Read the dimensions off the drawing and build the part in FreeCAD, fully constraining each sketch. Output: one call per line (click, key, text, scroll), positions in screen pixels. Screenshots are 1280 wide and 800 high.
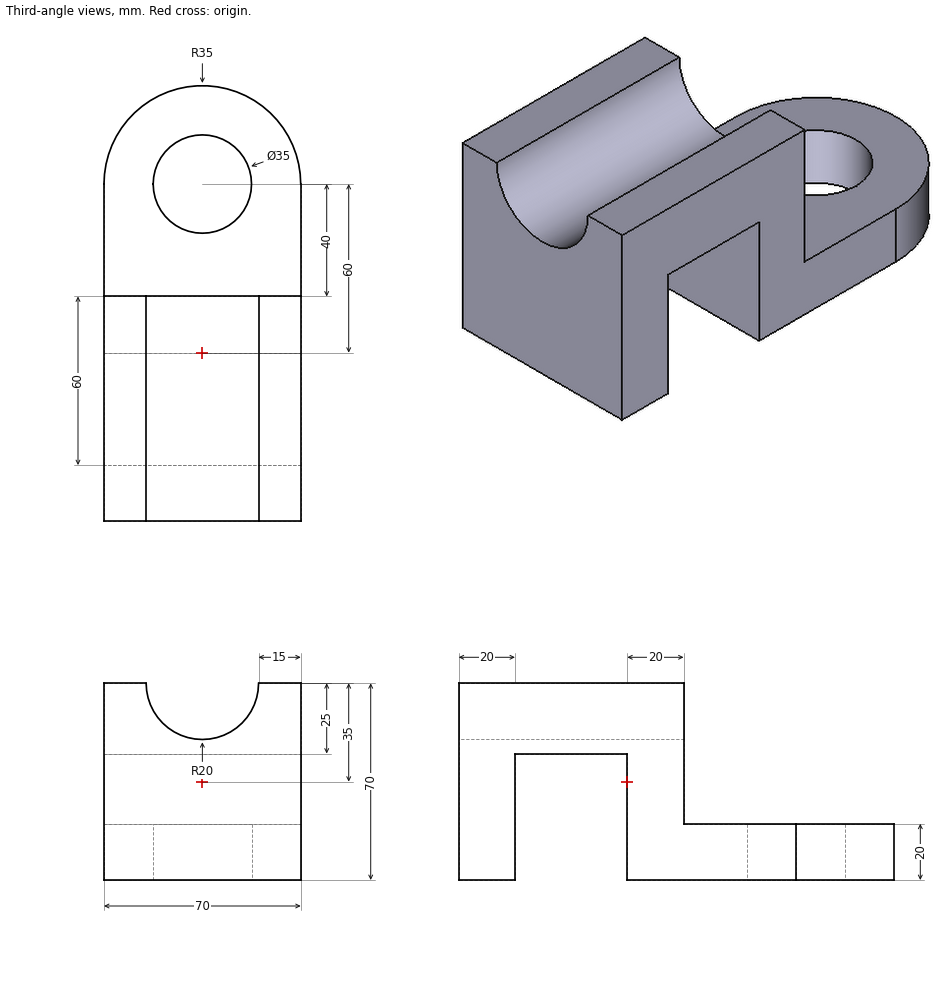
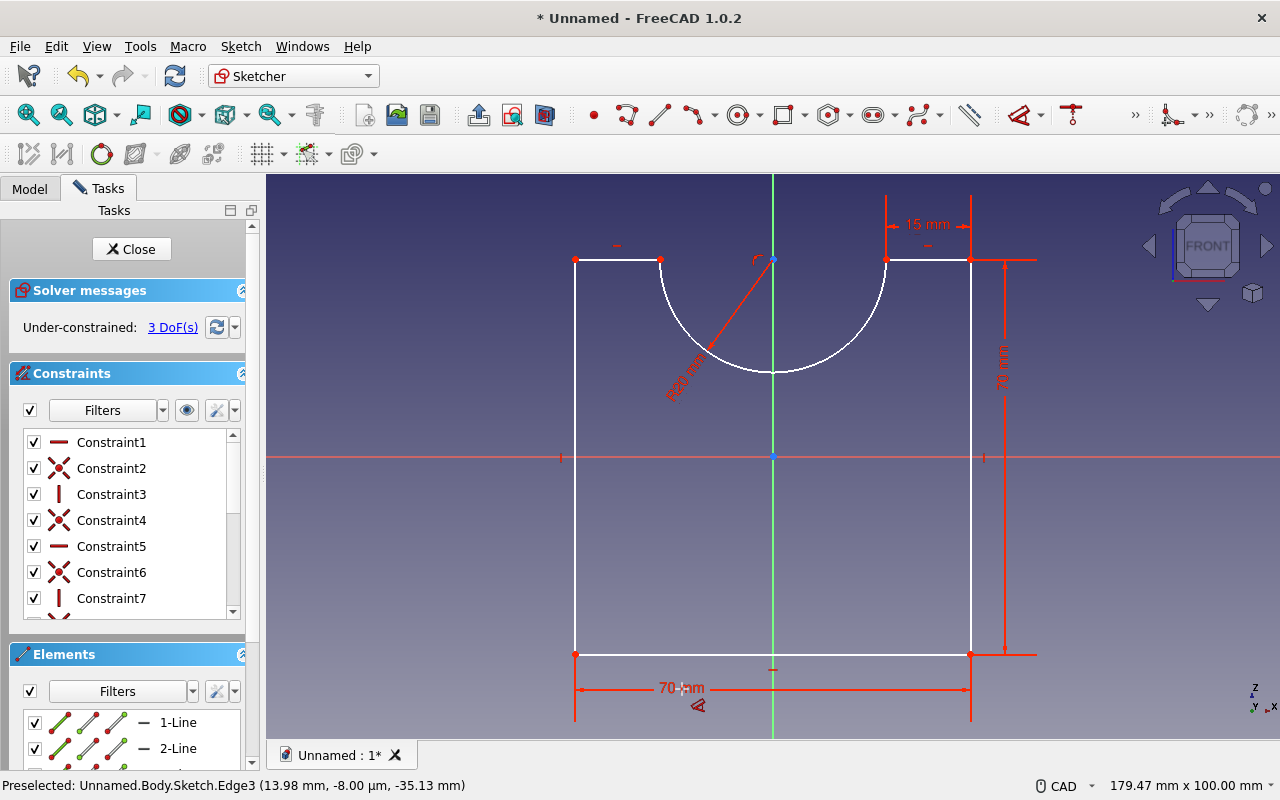
click(575, 536)
click(541, 367)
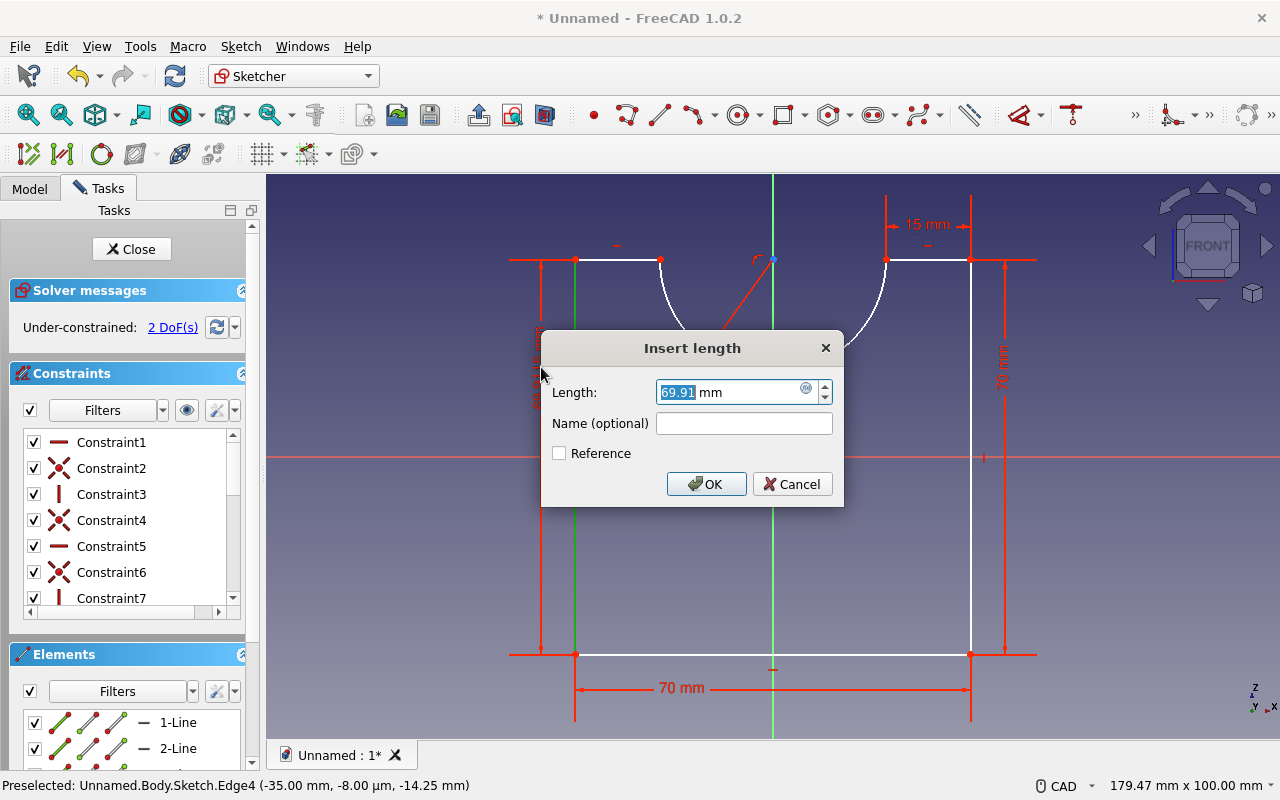
text(70)
key(Return)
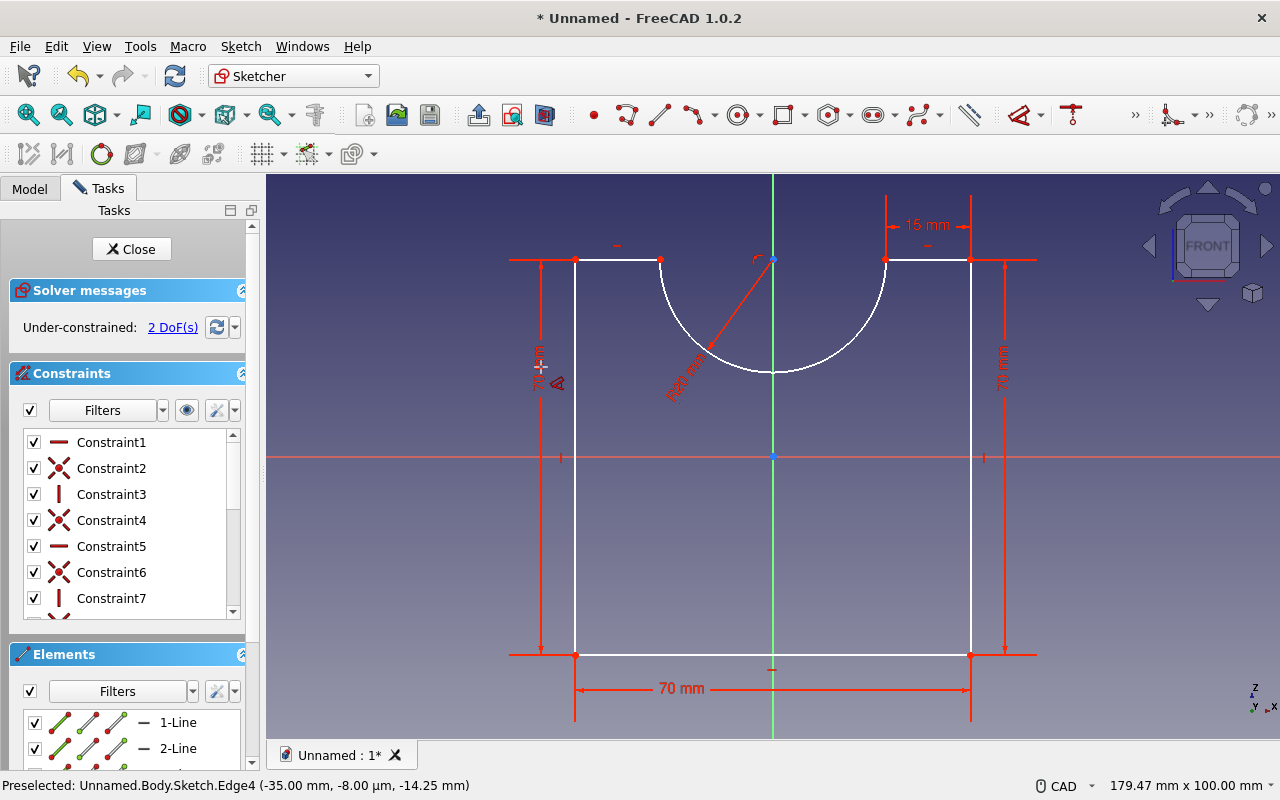
click(886, 260)
click(920, 358)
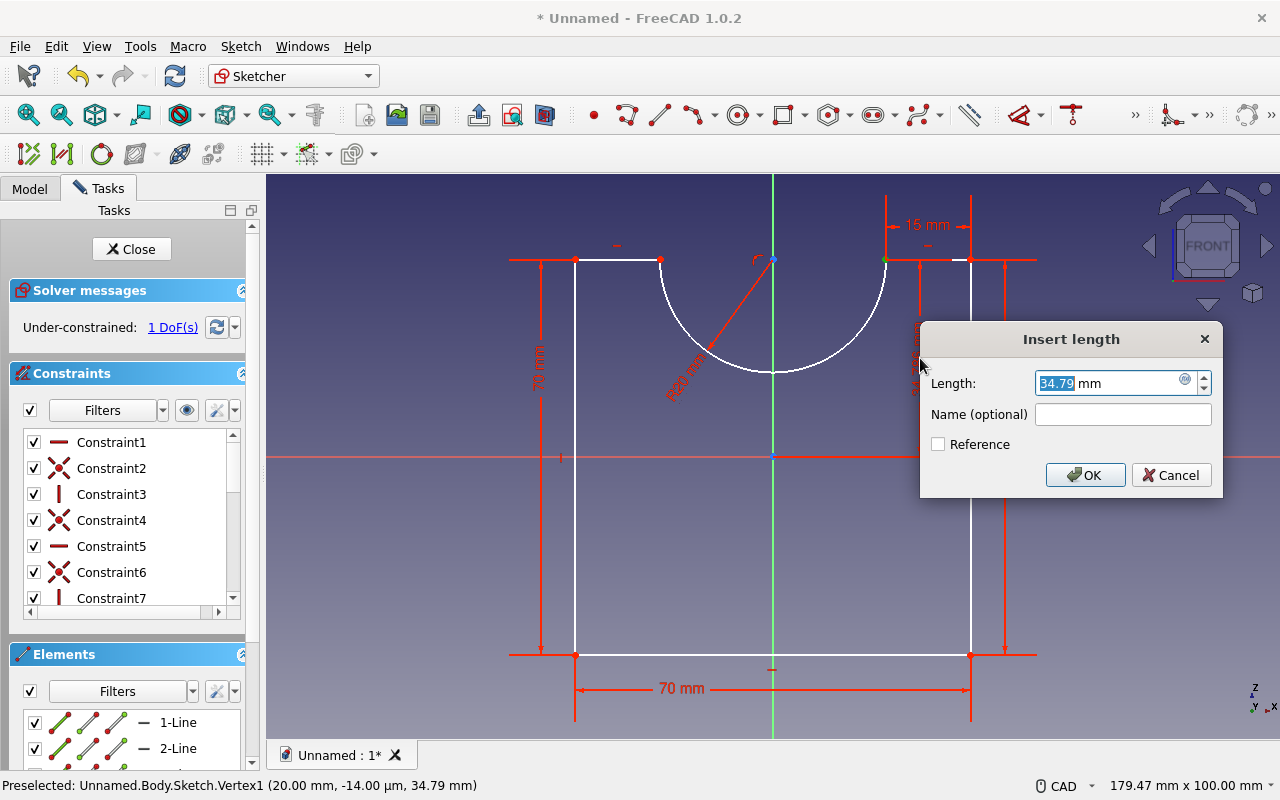
text(35)
key(Return)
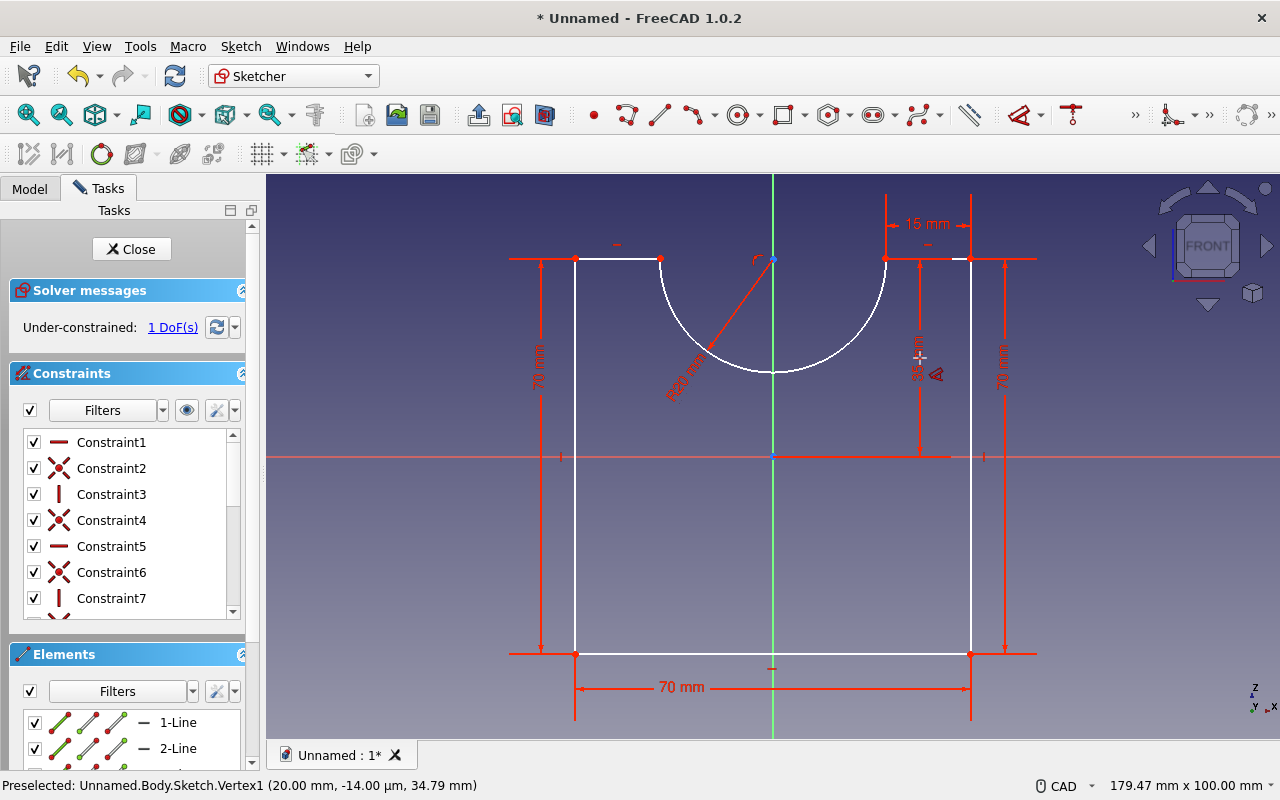
click(773, 260)
click(807, 313)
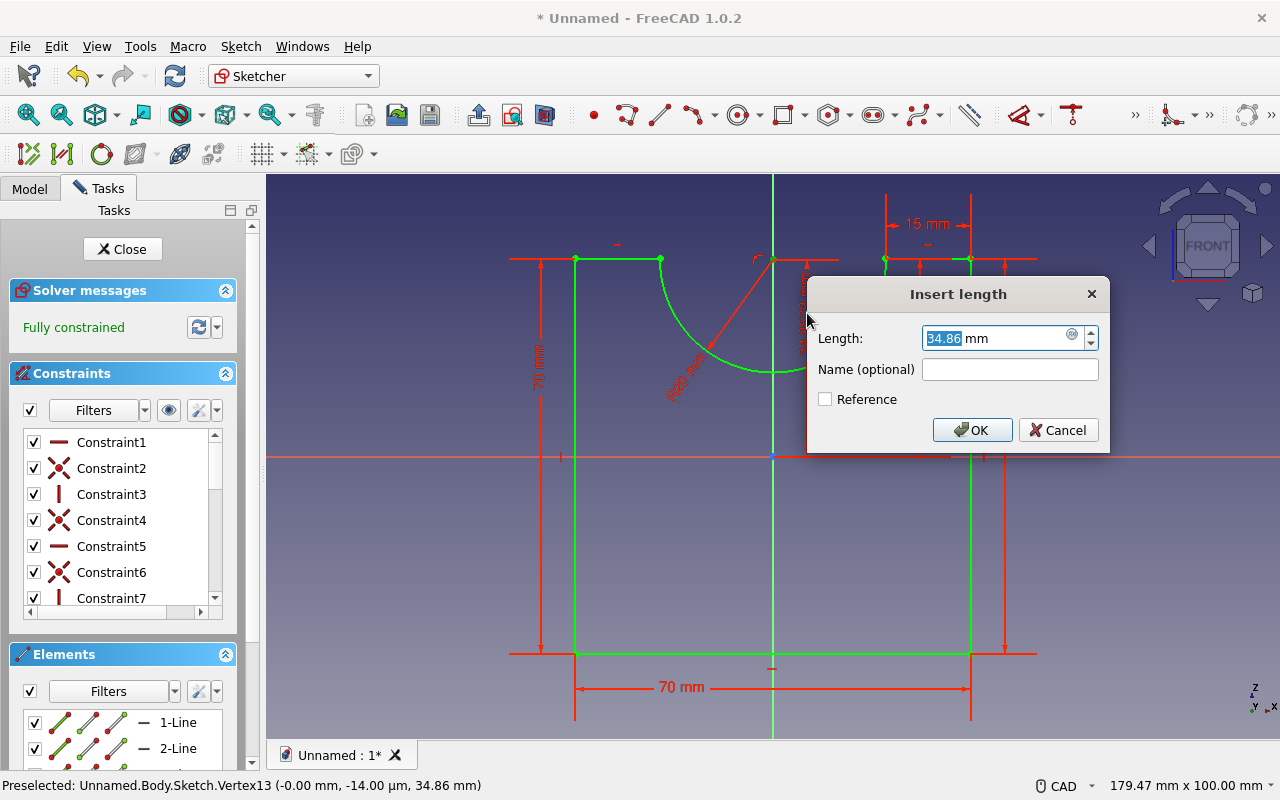
text(35)
key(Return)
key(Escape)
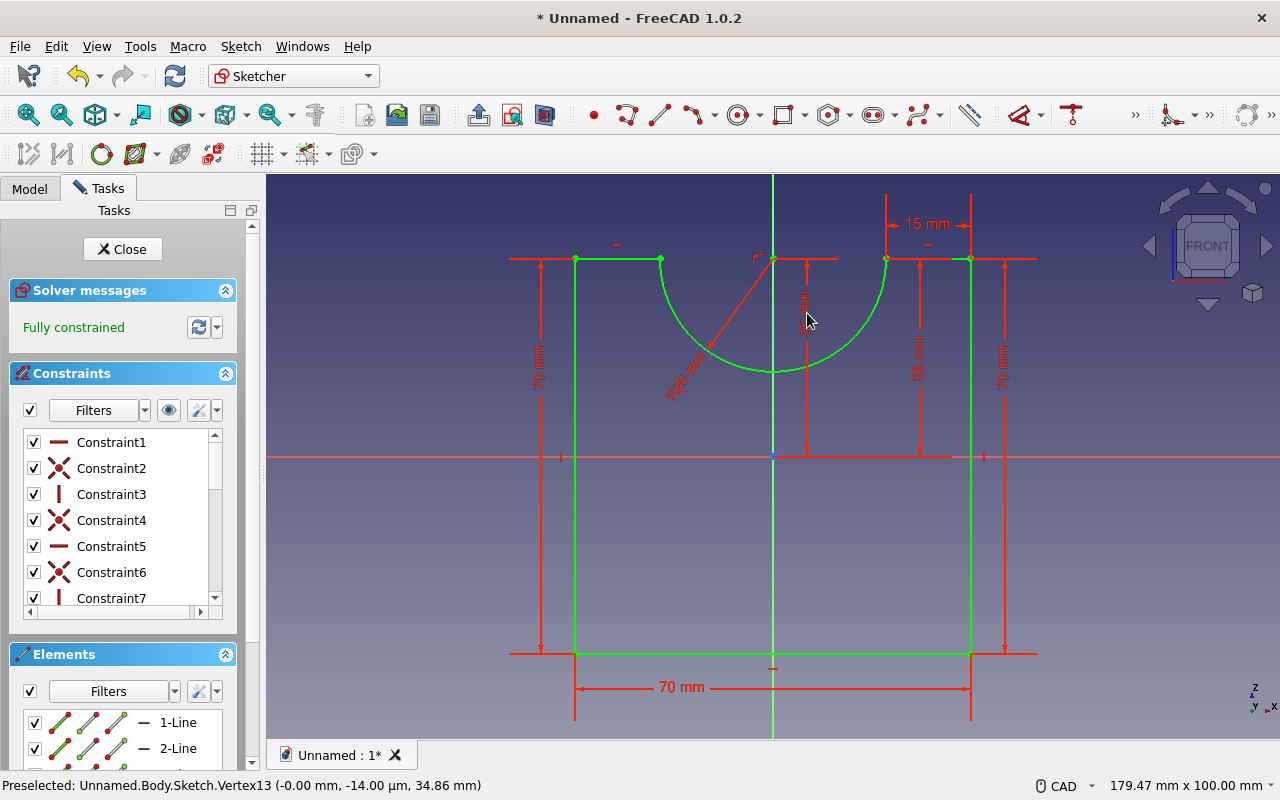
click(123, 249)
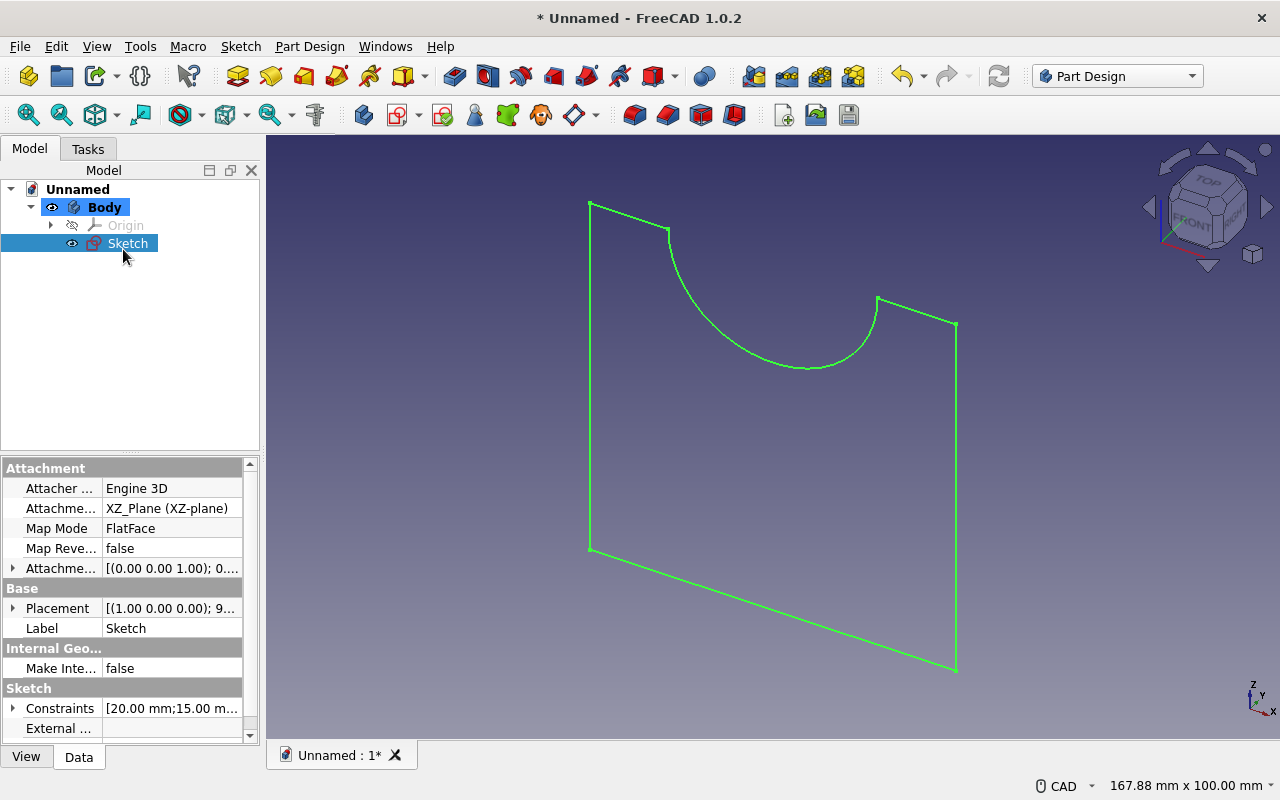
click(238, 76)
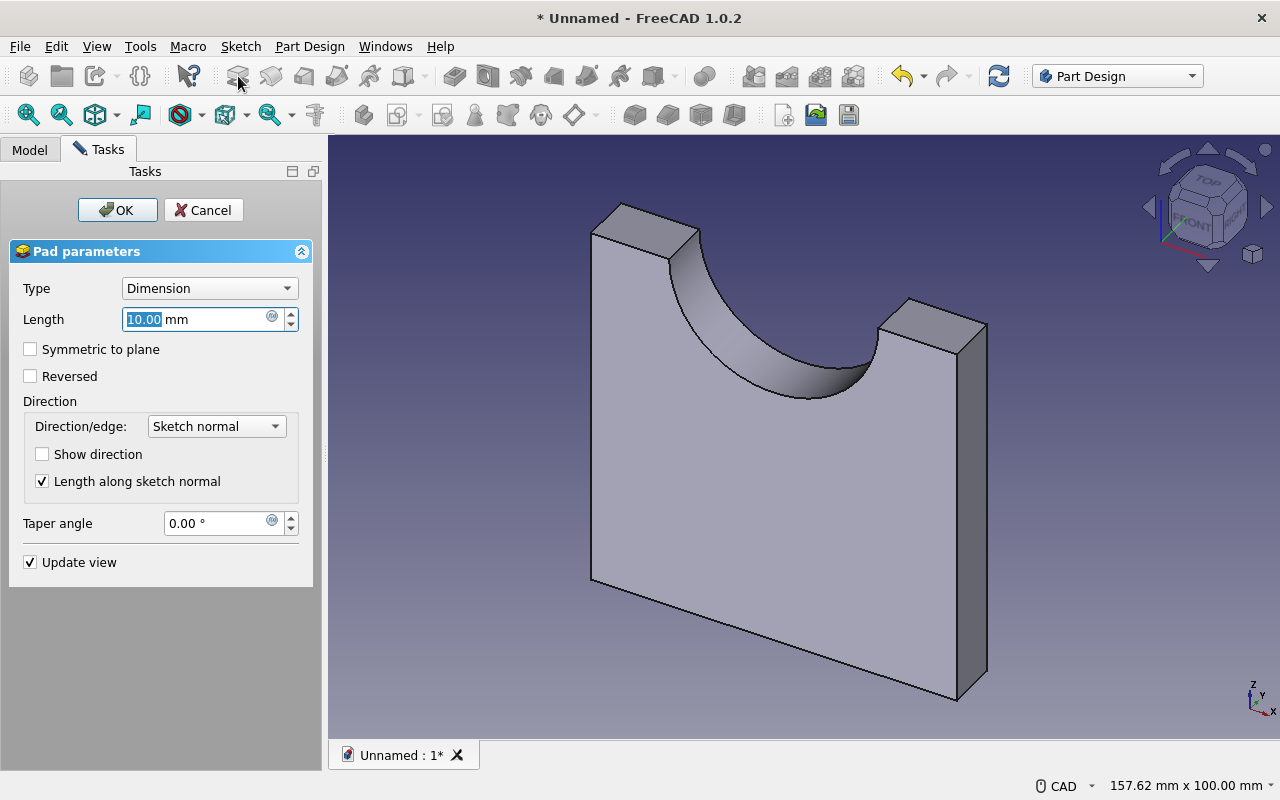
text(20)
key(Tab)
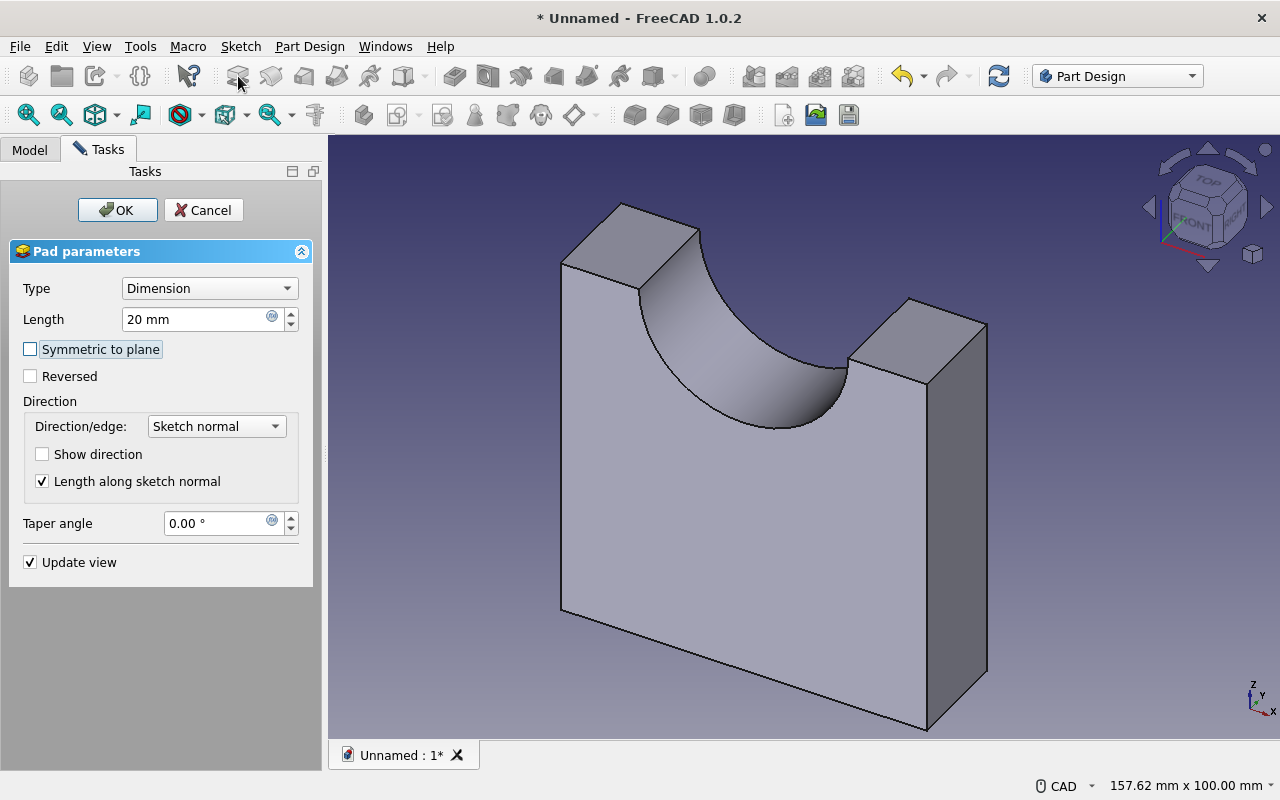
click(31, 376)